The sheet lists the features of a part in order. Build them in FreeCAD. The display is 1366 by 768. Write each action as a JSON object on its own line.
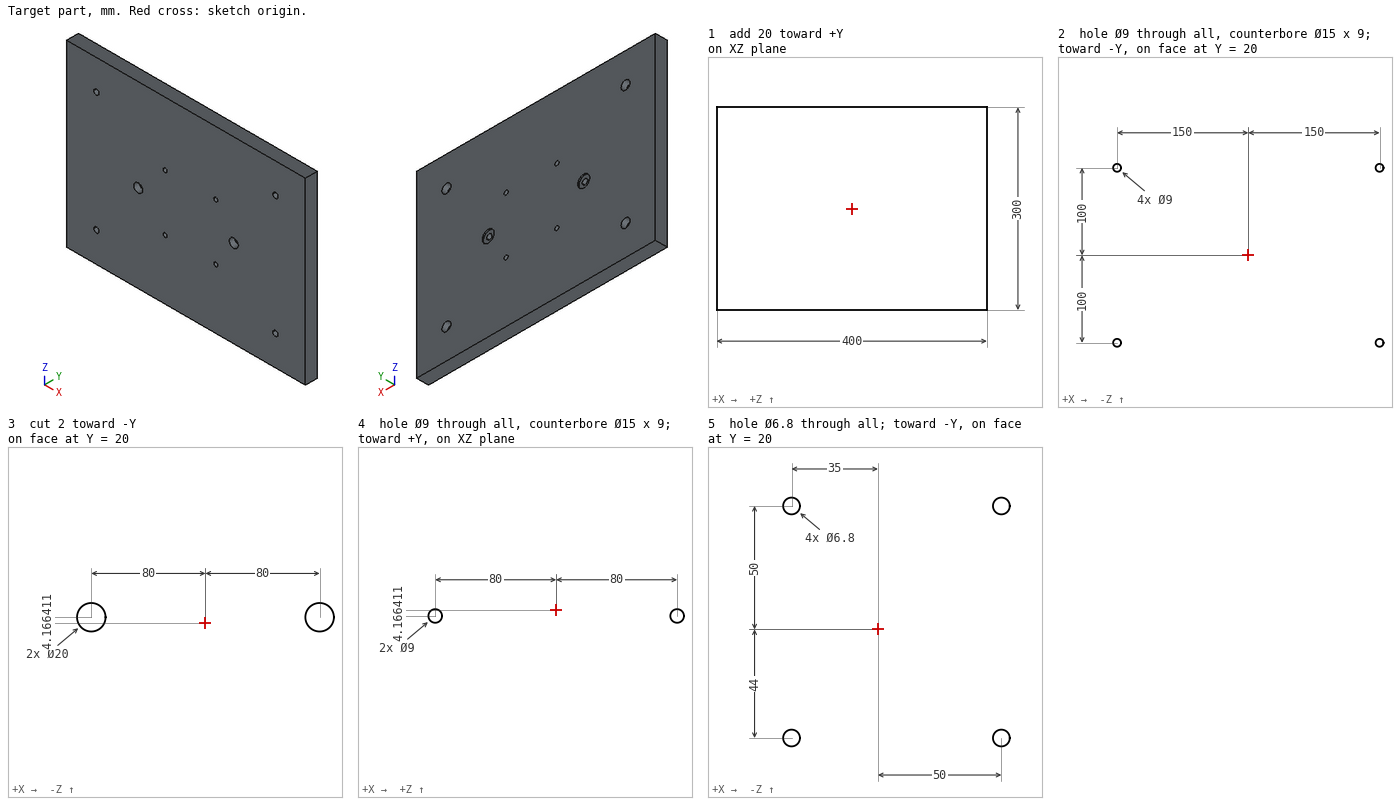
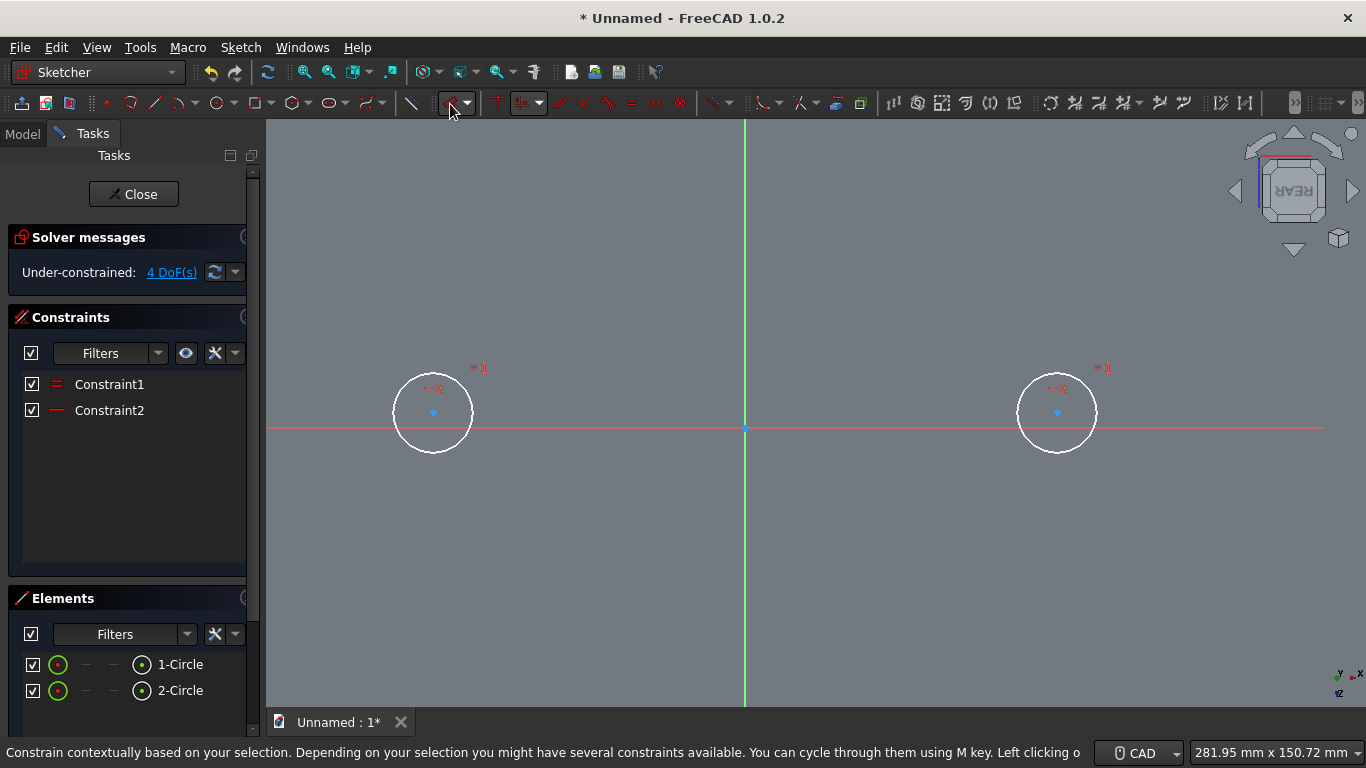
{"action": "left_click", "coordinate": [461, 385]}
{"action": "left_click", "coordinate": [484, 362]}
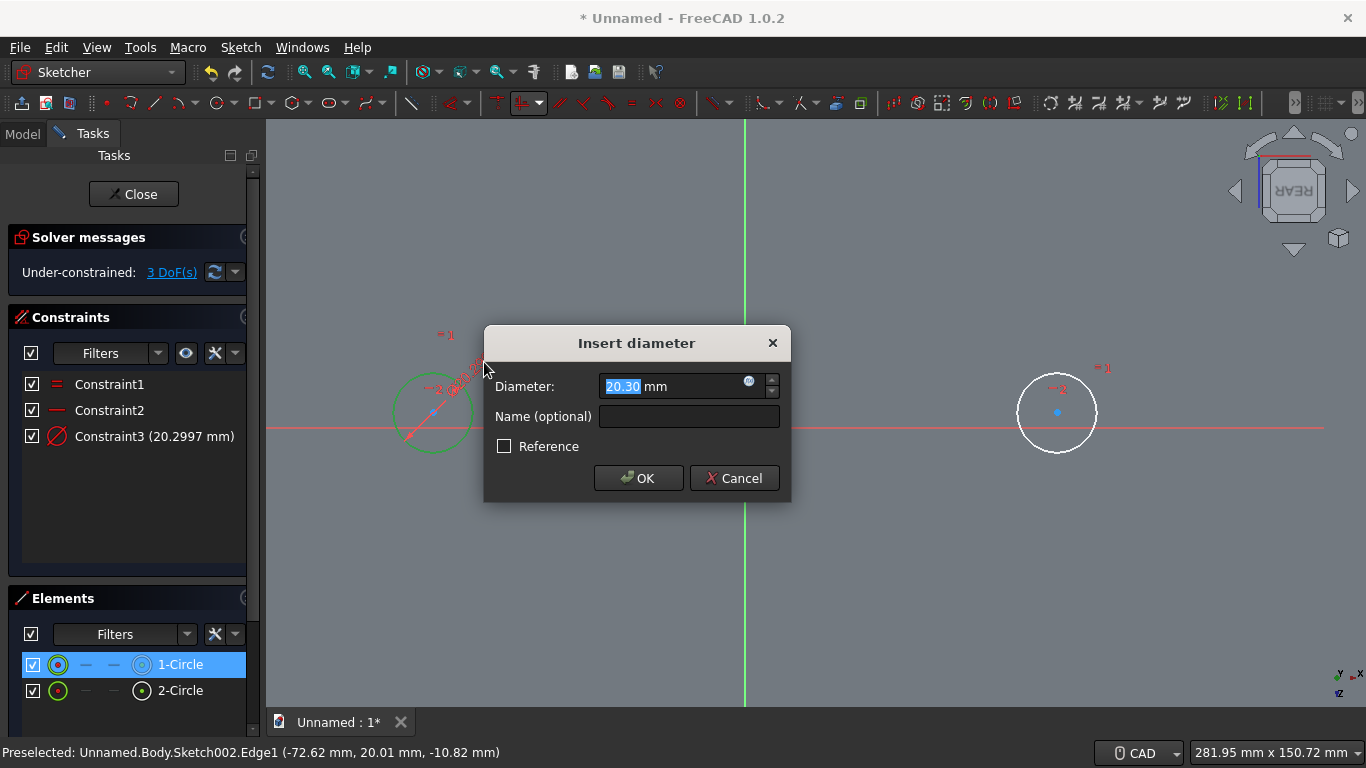
{"action": "type", "text": "20"}
{"action": "key", "text": "Return"}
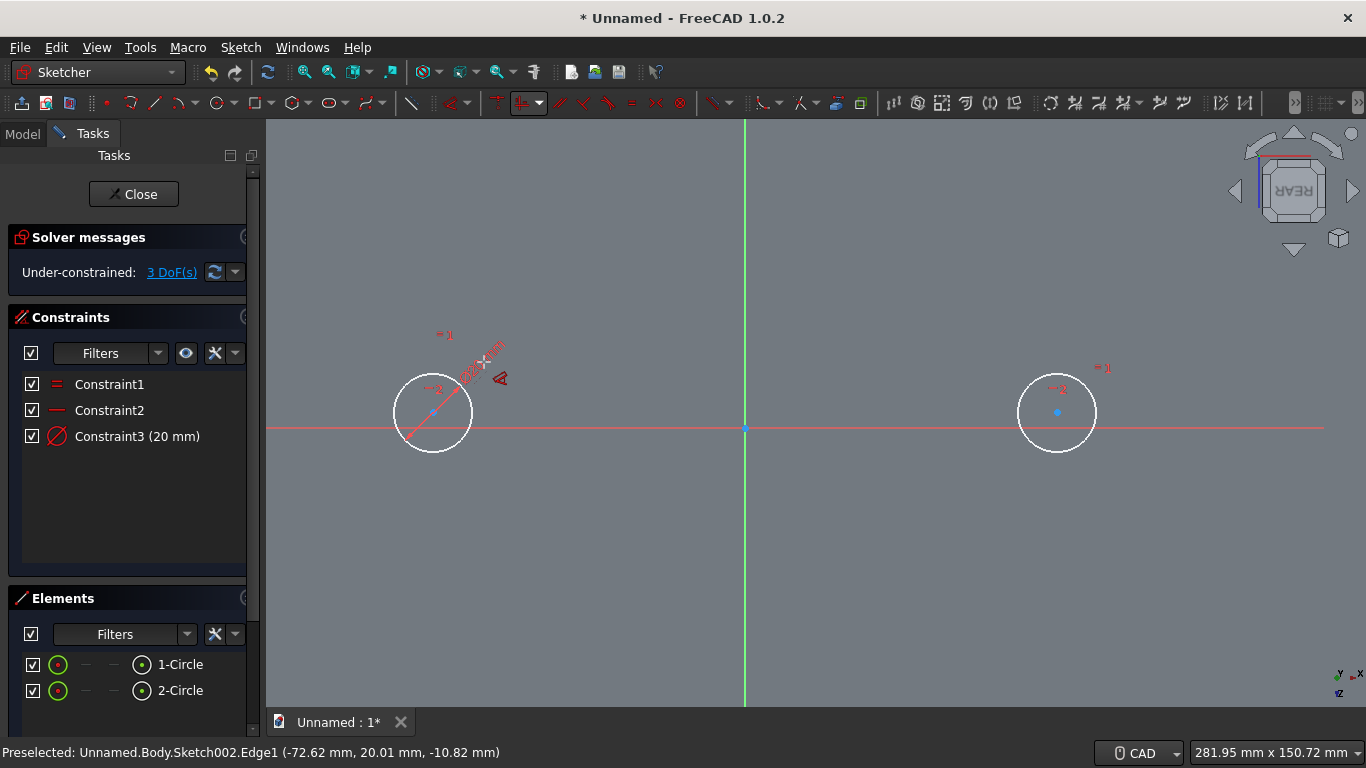
{"action": "left_click", "coordinate": [433, 413]}
{"action": "left_click", "coordinate": [589, 462]}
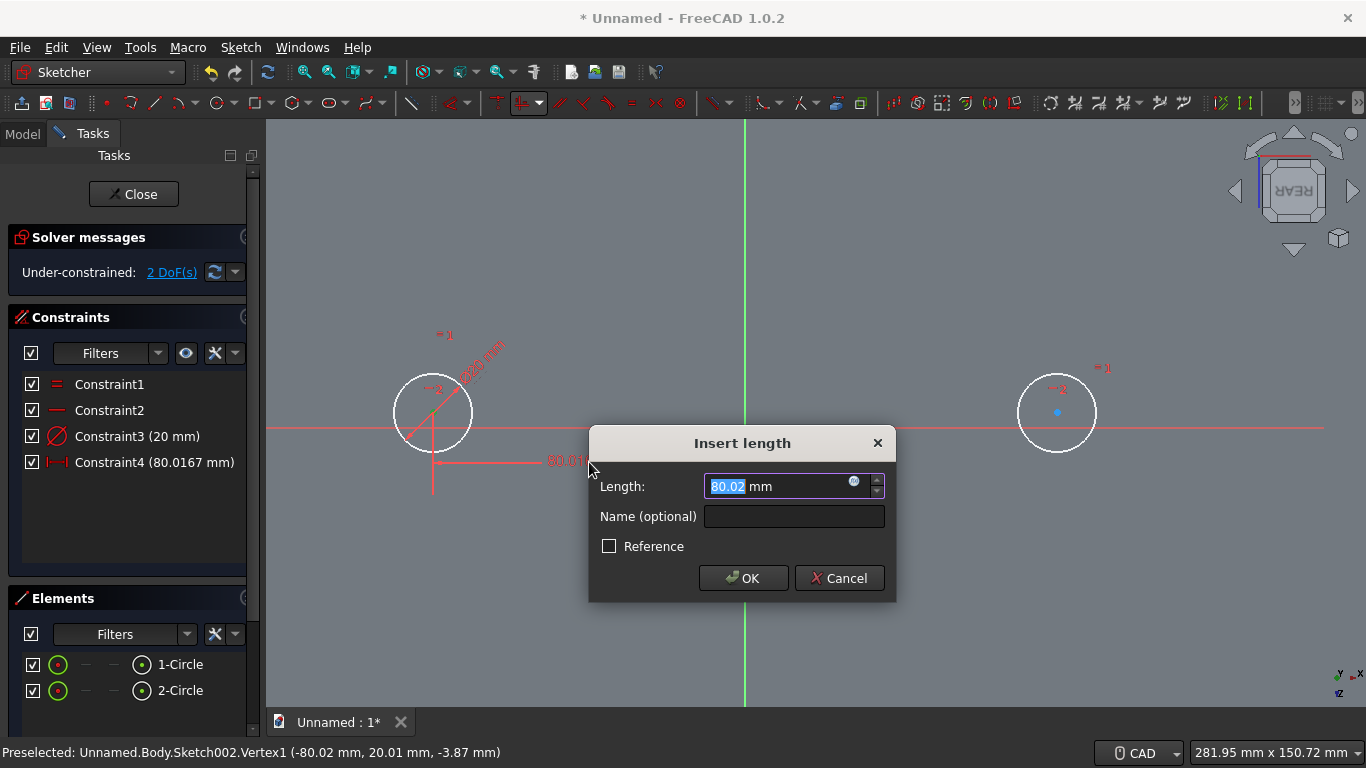
{"action": "type", "text": "80"}
{"action": "key", "text": "Return"}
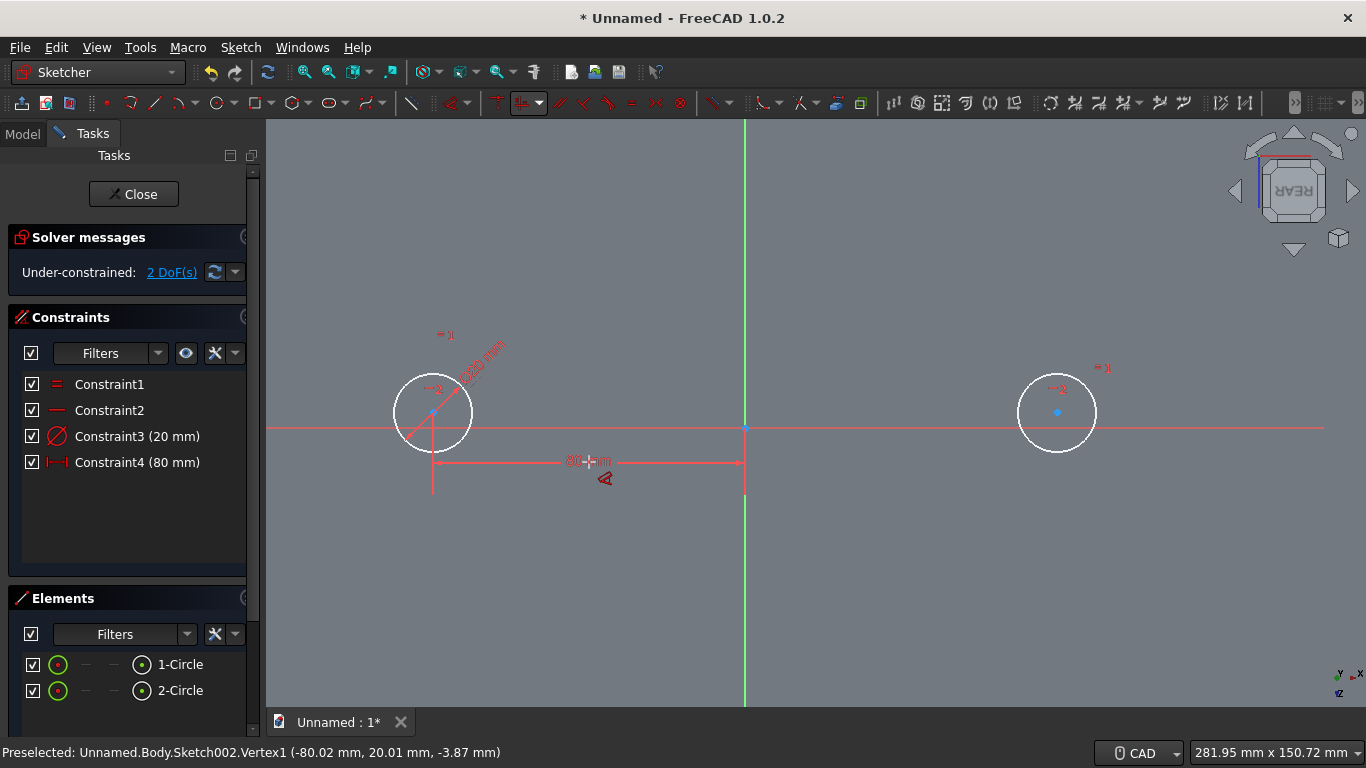
{"action": "left_click", "coordinate": [1057, 413]}
{"action": "left_click", "coordinate": [901, 462]}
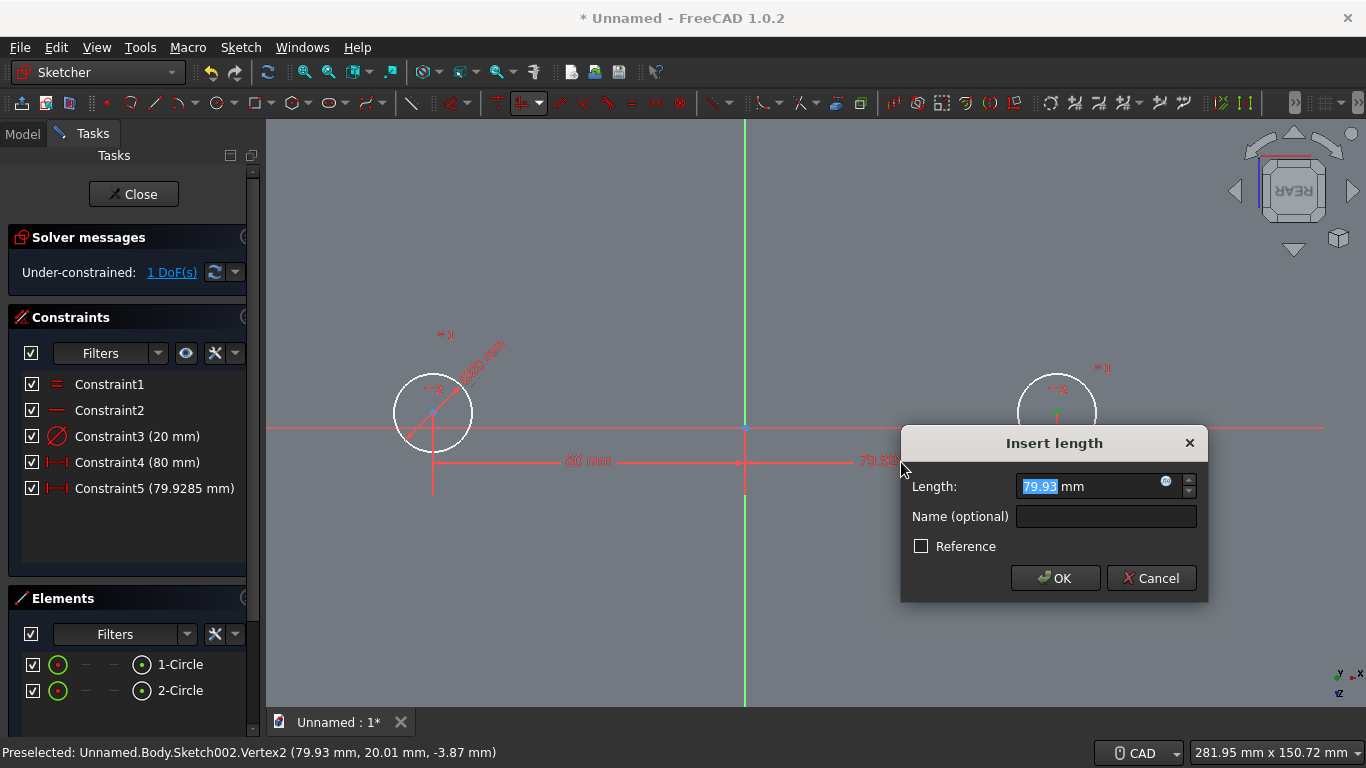
{"action": "type", "text": "80"}
{"action": "key", "text": "Return"}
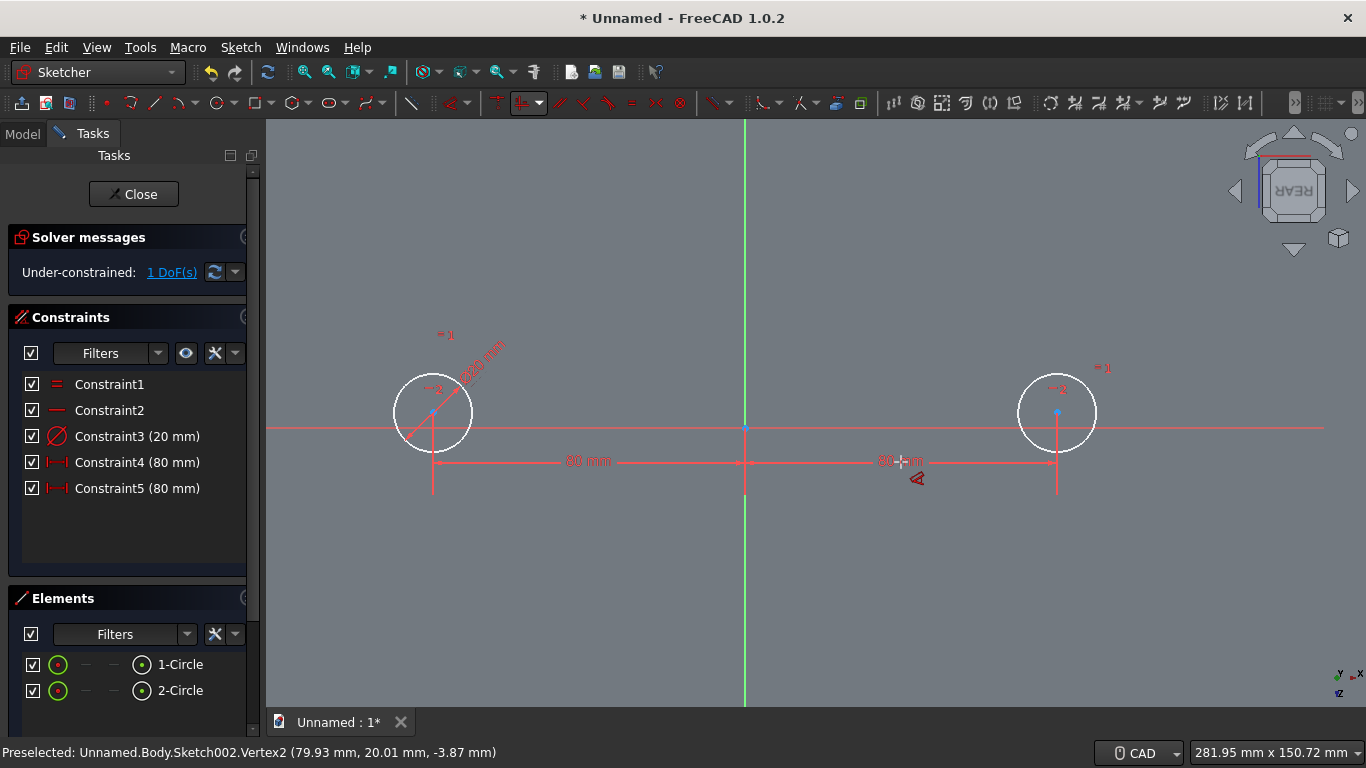
{"action": "scroll", "coordinate": [433, 413], "scroll_direction": "up", "scroll_amount": 5}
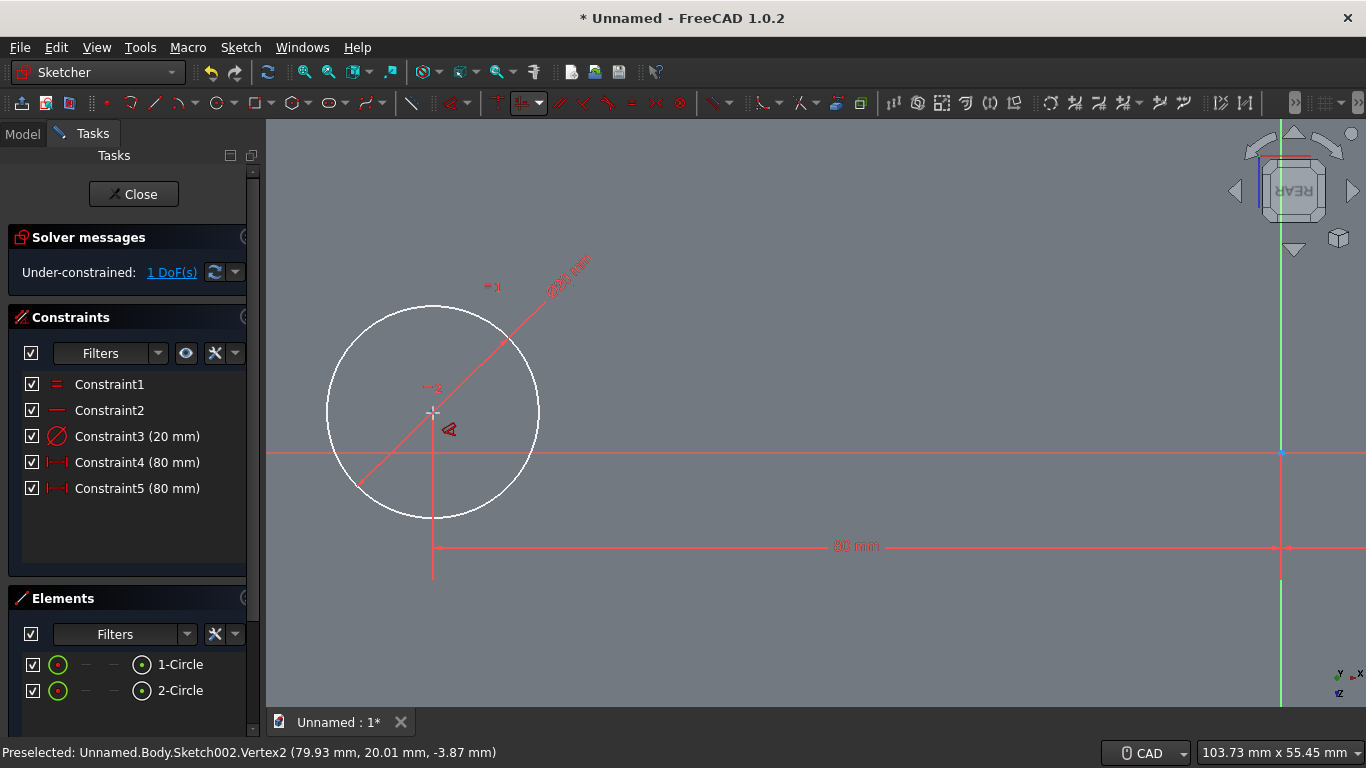
{"action": "left_click", "coordinate": [433, 412]}
{"action": "left_click", "coordinate": [399, 433]}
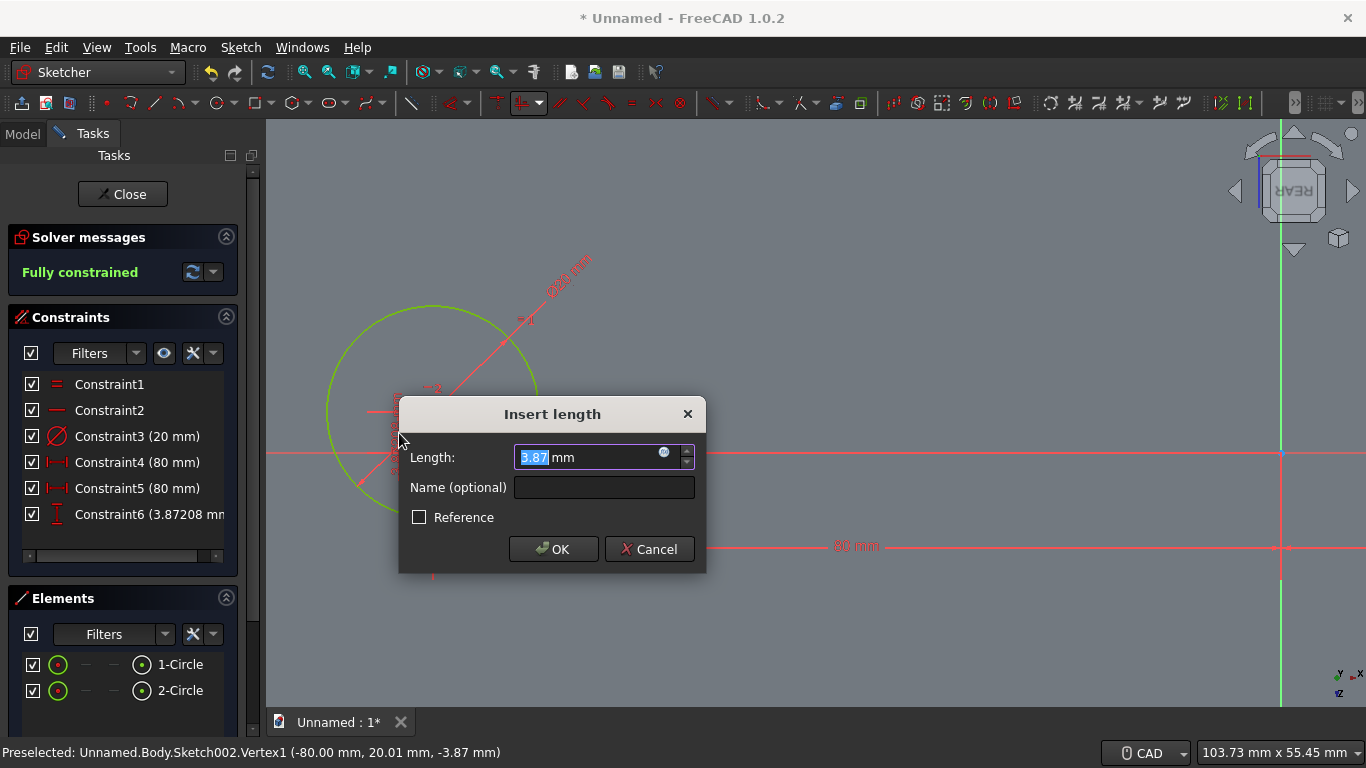
{"action": "type", "text": "4.166411"}
{"action": "key", "text": "Return"}
{"action": "key", "text": "Escape"}